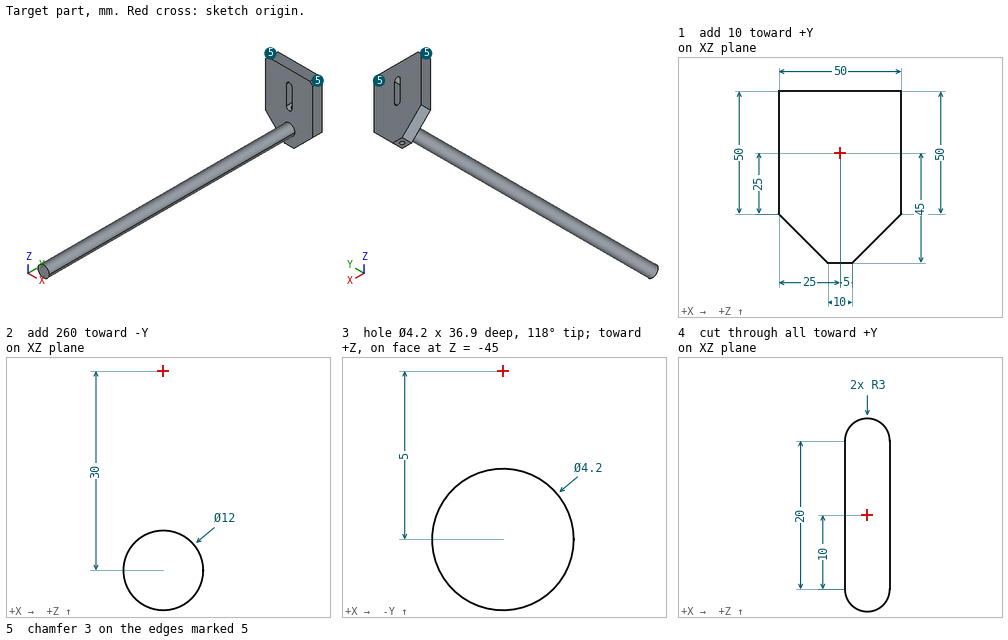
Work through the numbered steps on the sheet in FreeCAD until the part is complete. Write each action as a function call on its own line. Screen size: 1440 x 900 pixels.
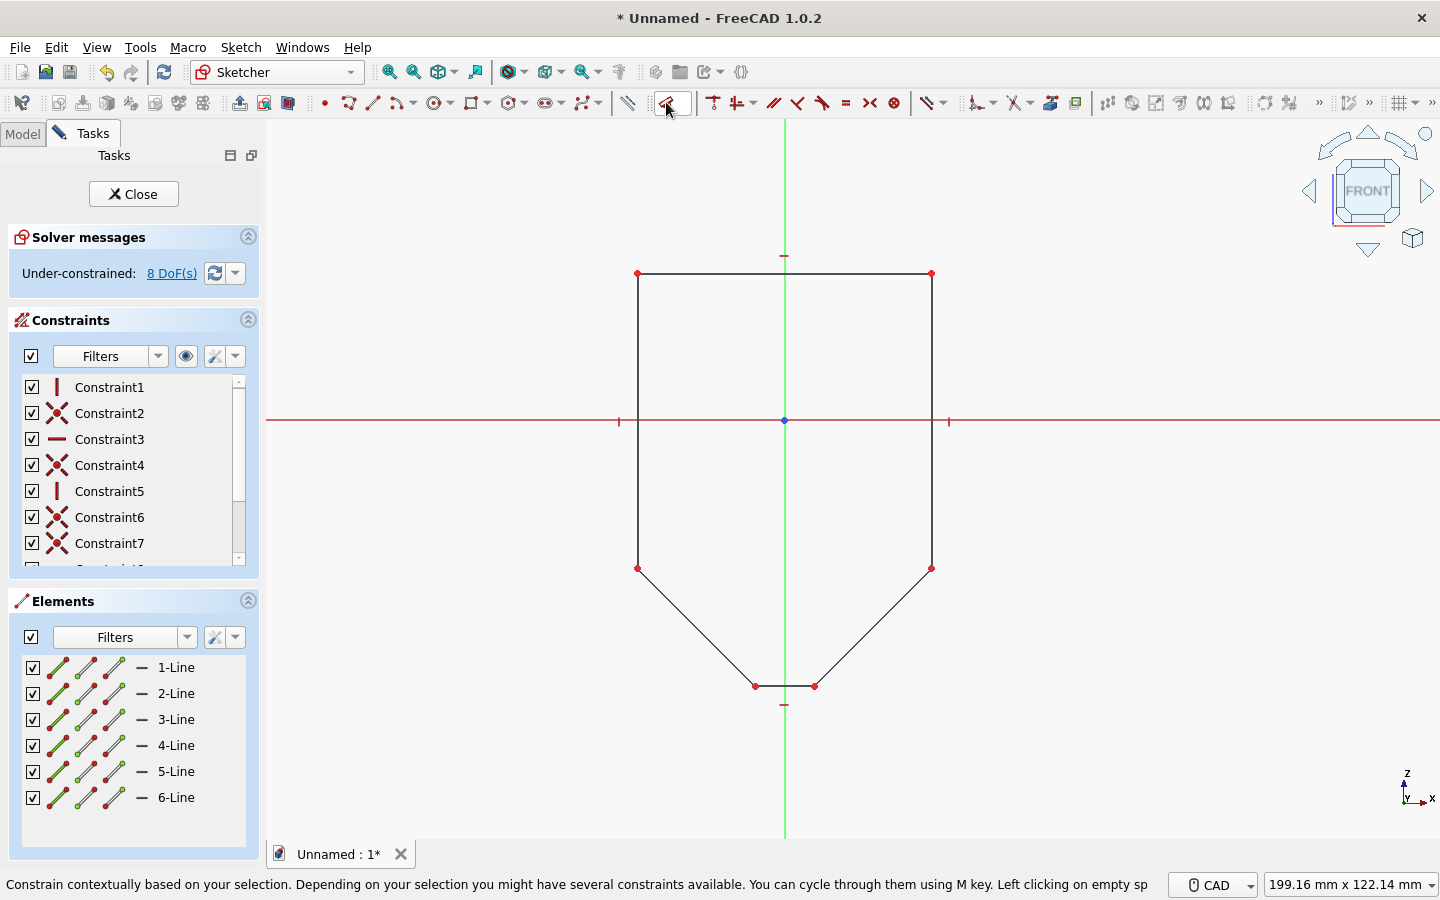
click(638, 480)
click(604, 353)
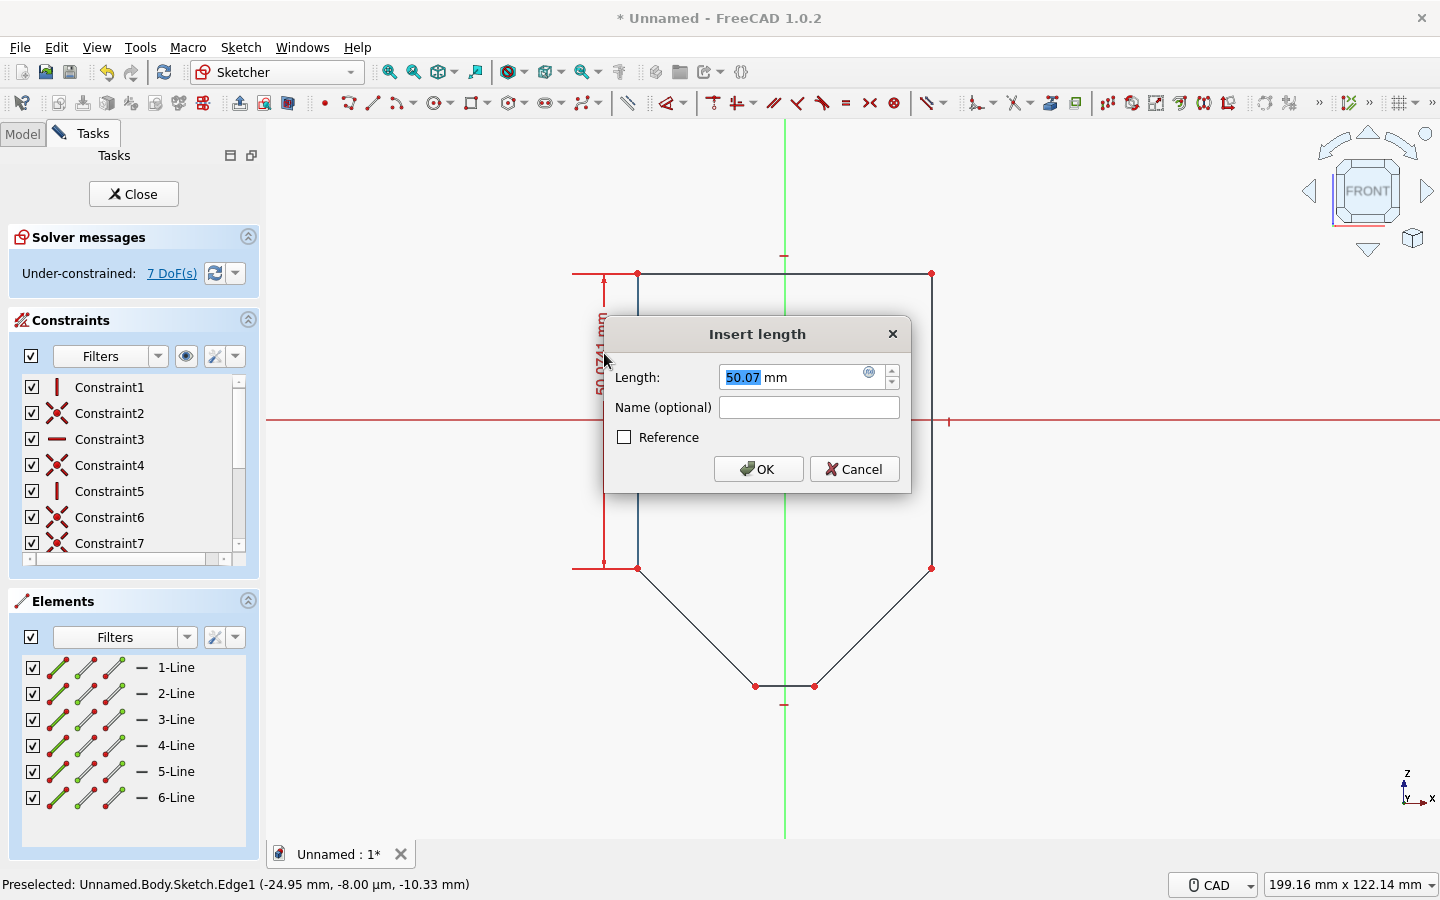
text(50)
key(Return)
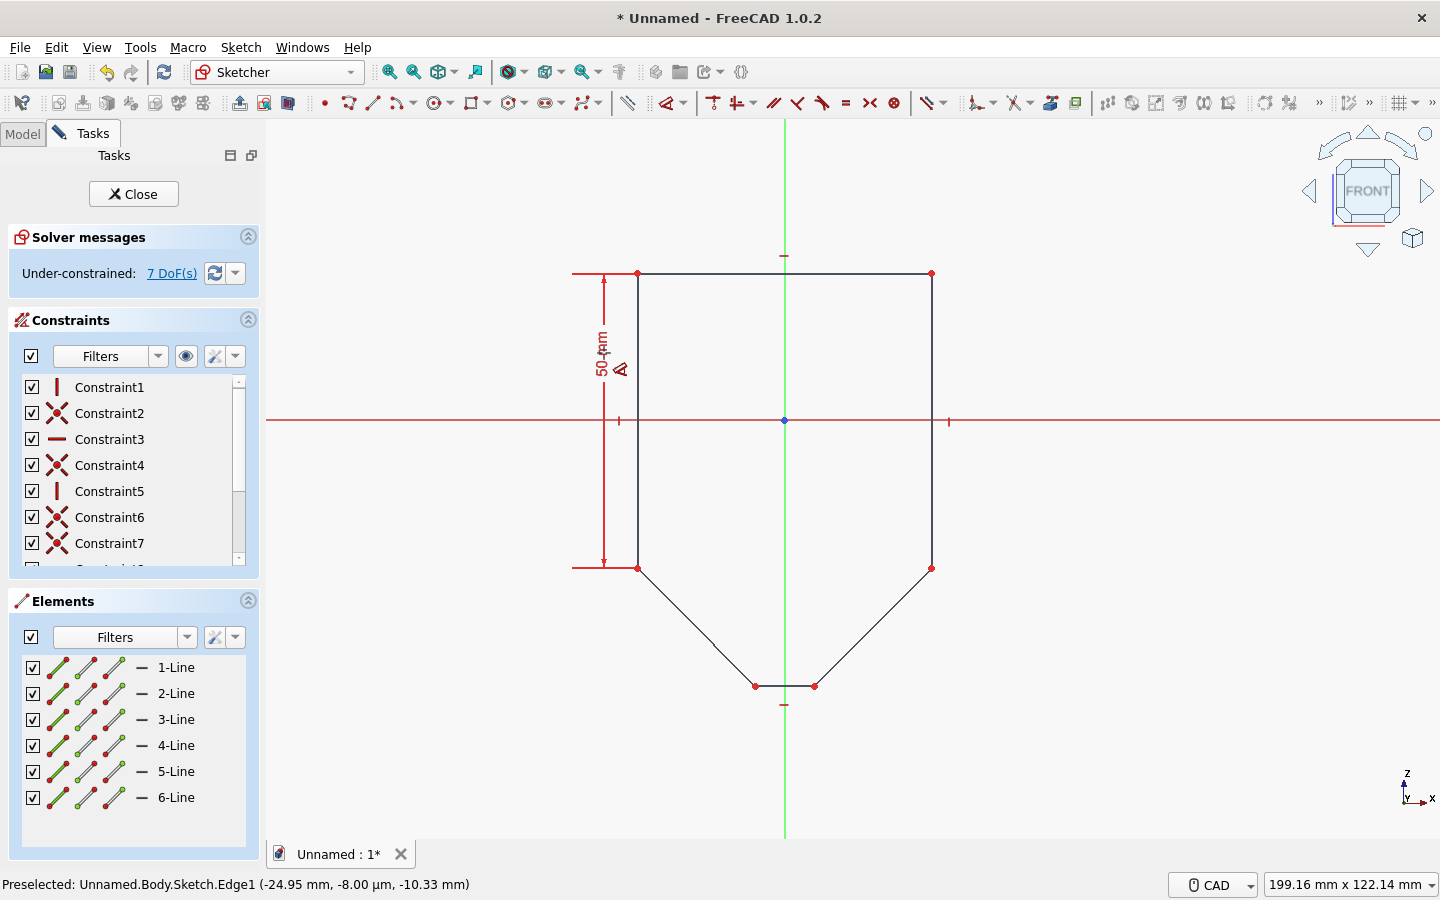
click(726, 274)
click(717, 240)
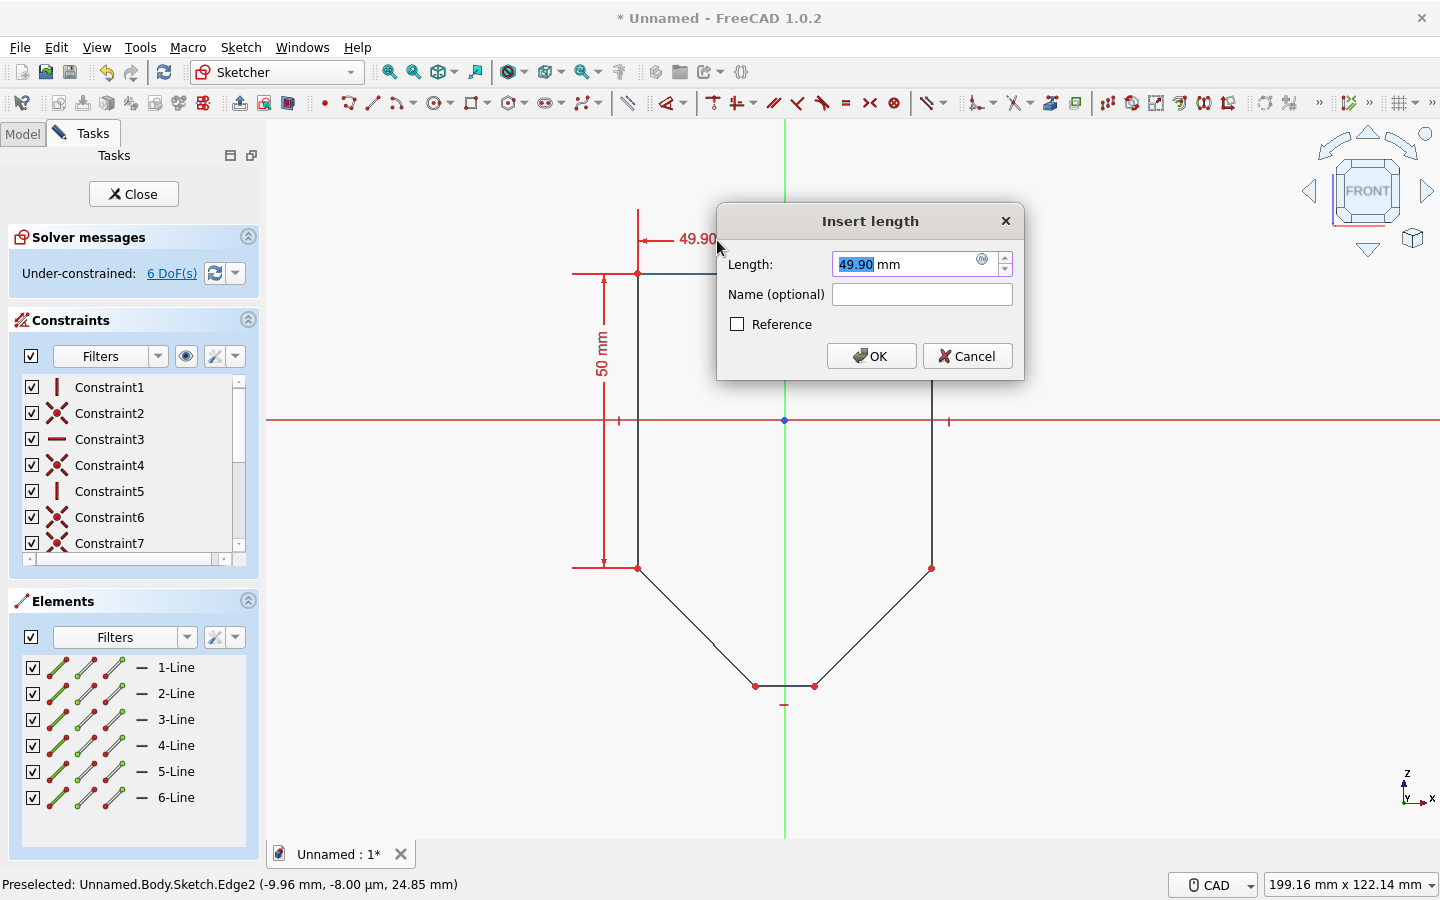
text(50)
key(Return)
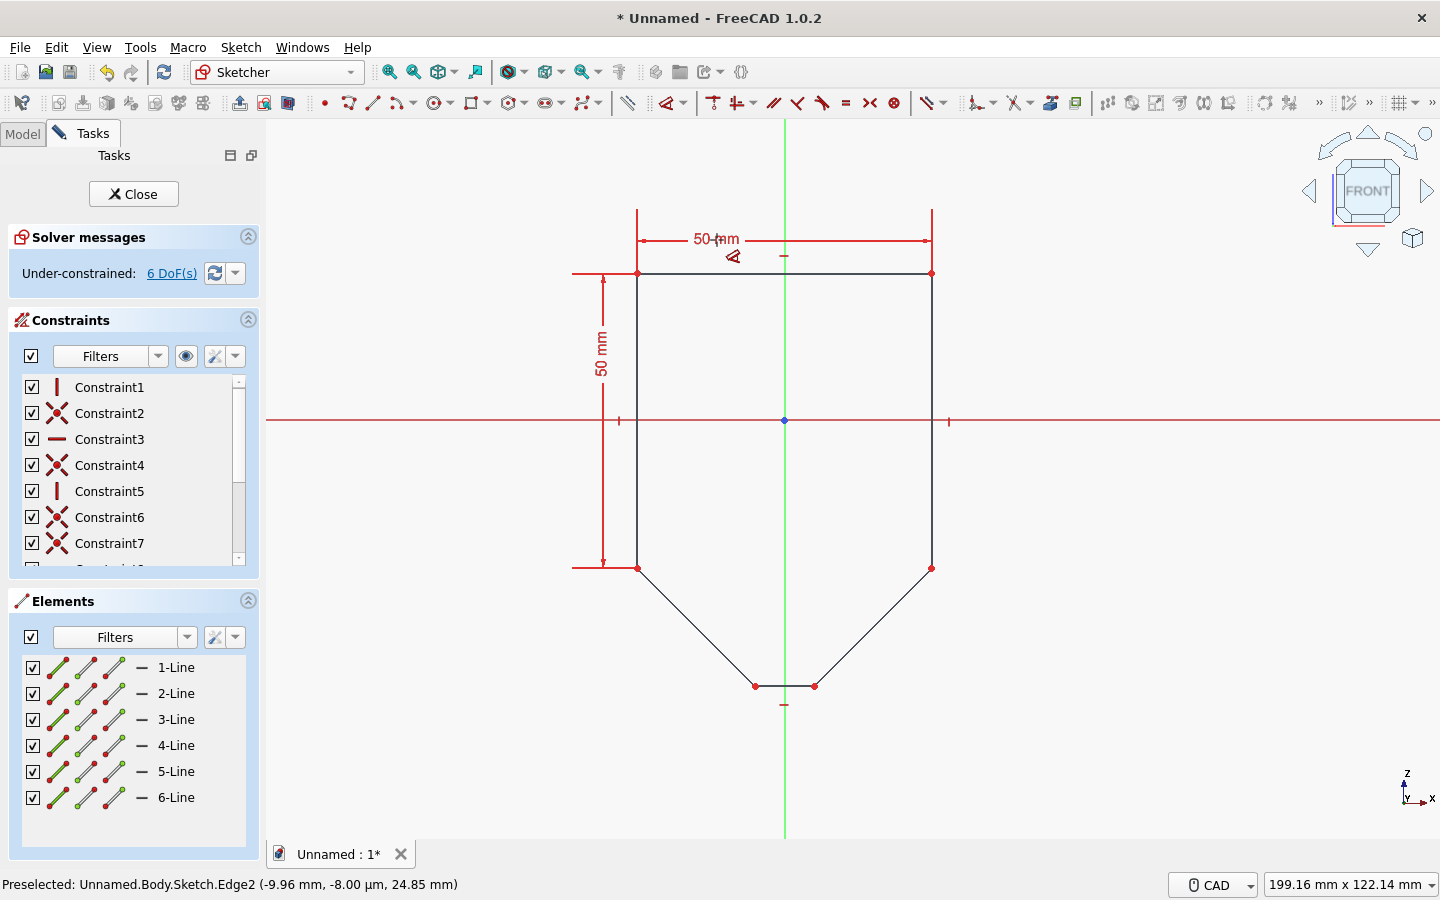
click(932, 362)
click(966, 353)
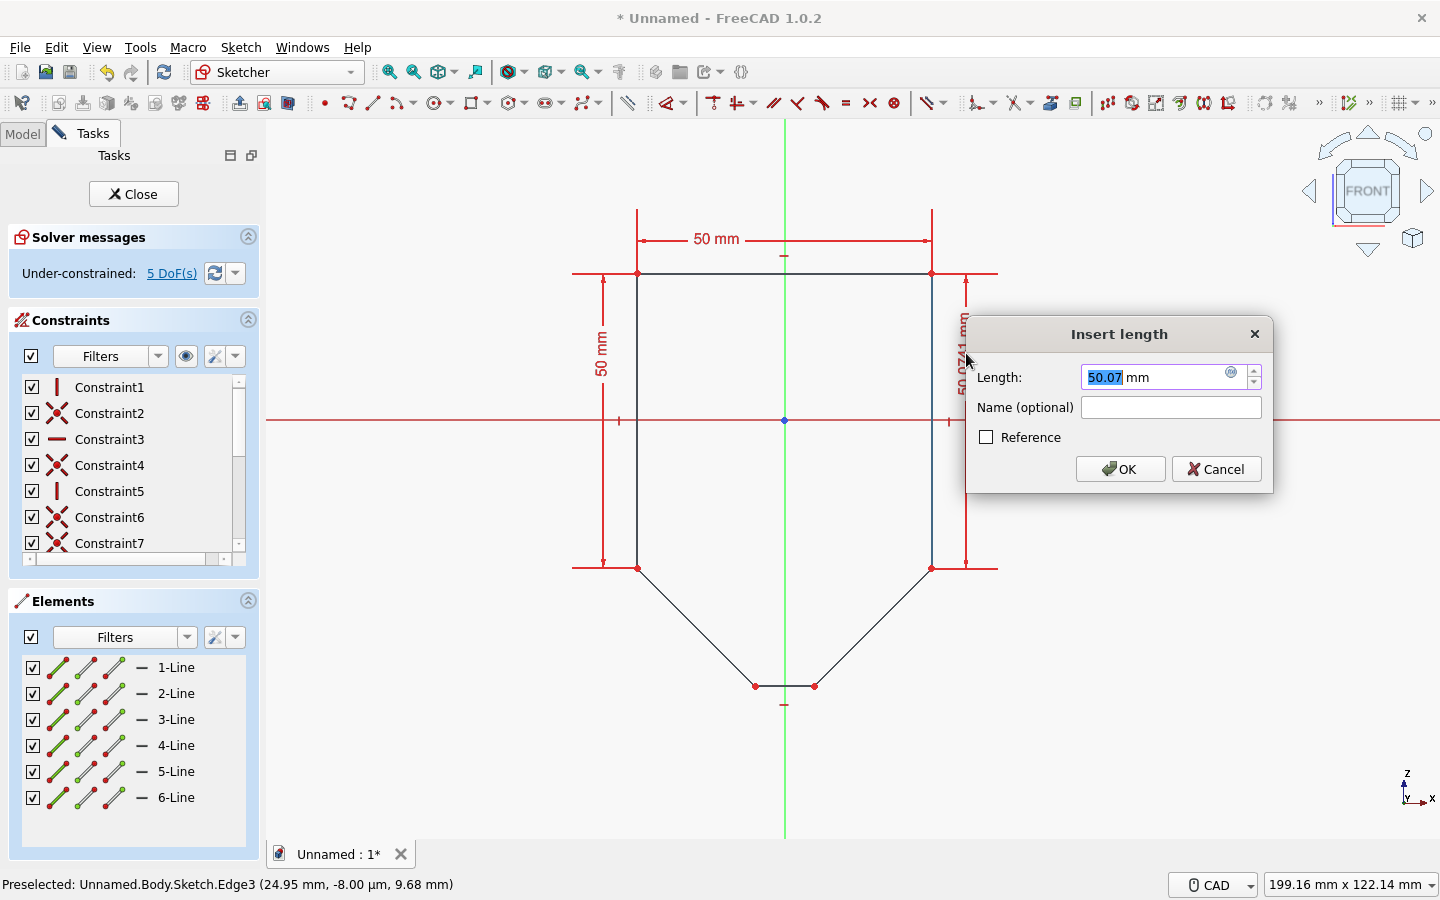
text(50)
key(Return)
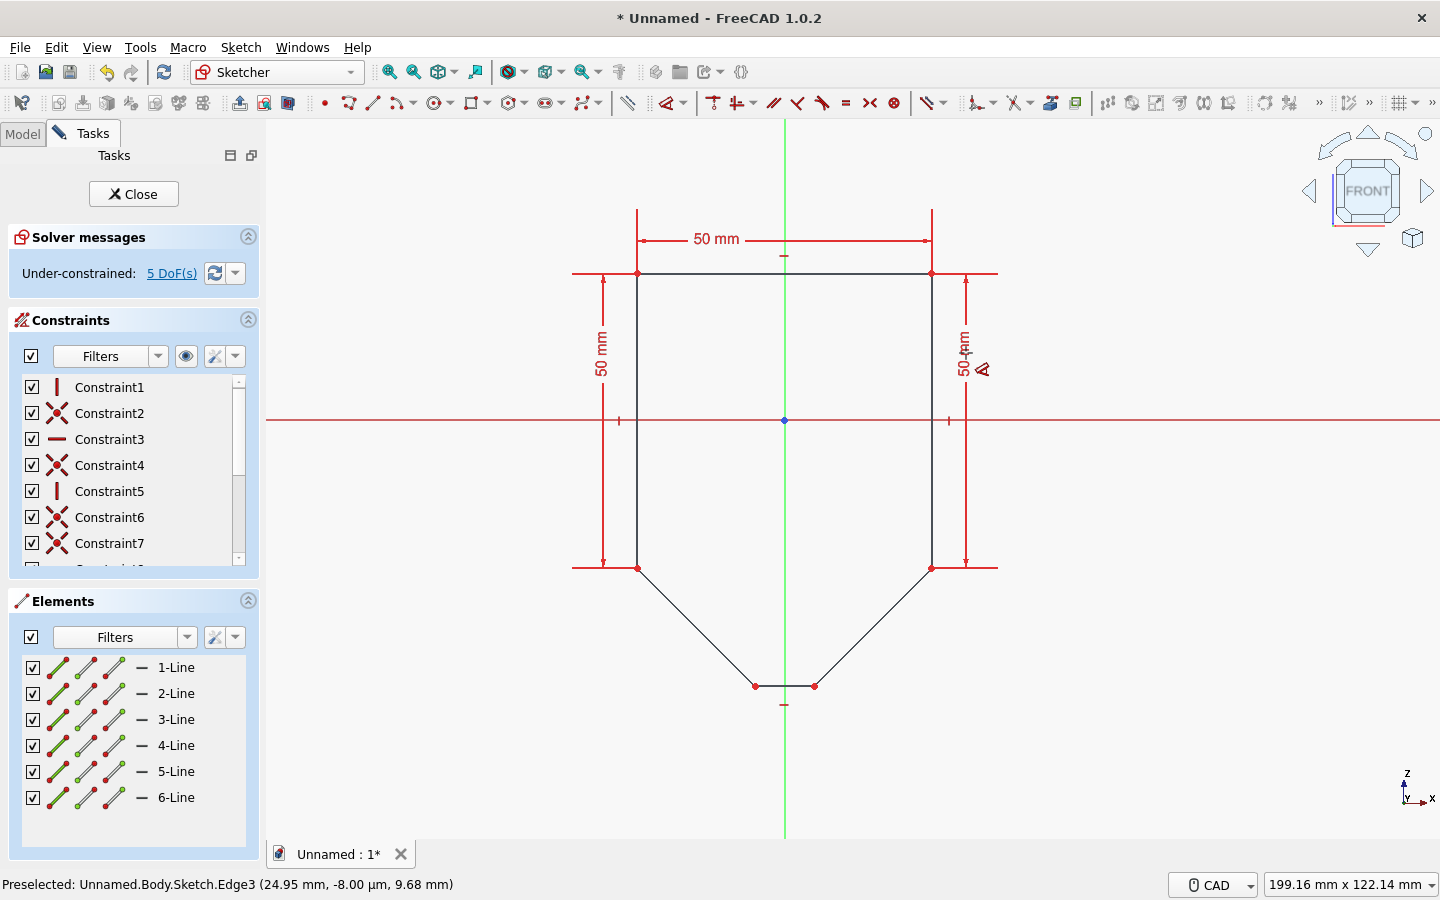
click(796, 686)
click(771, 720)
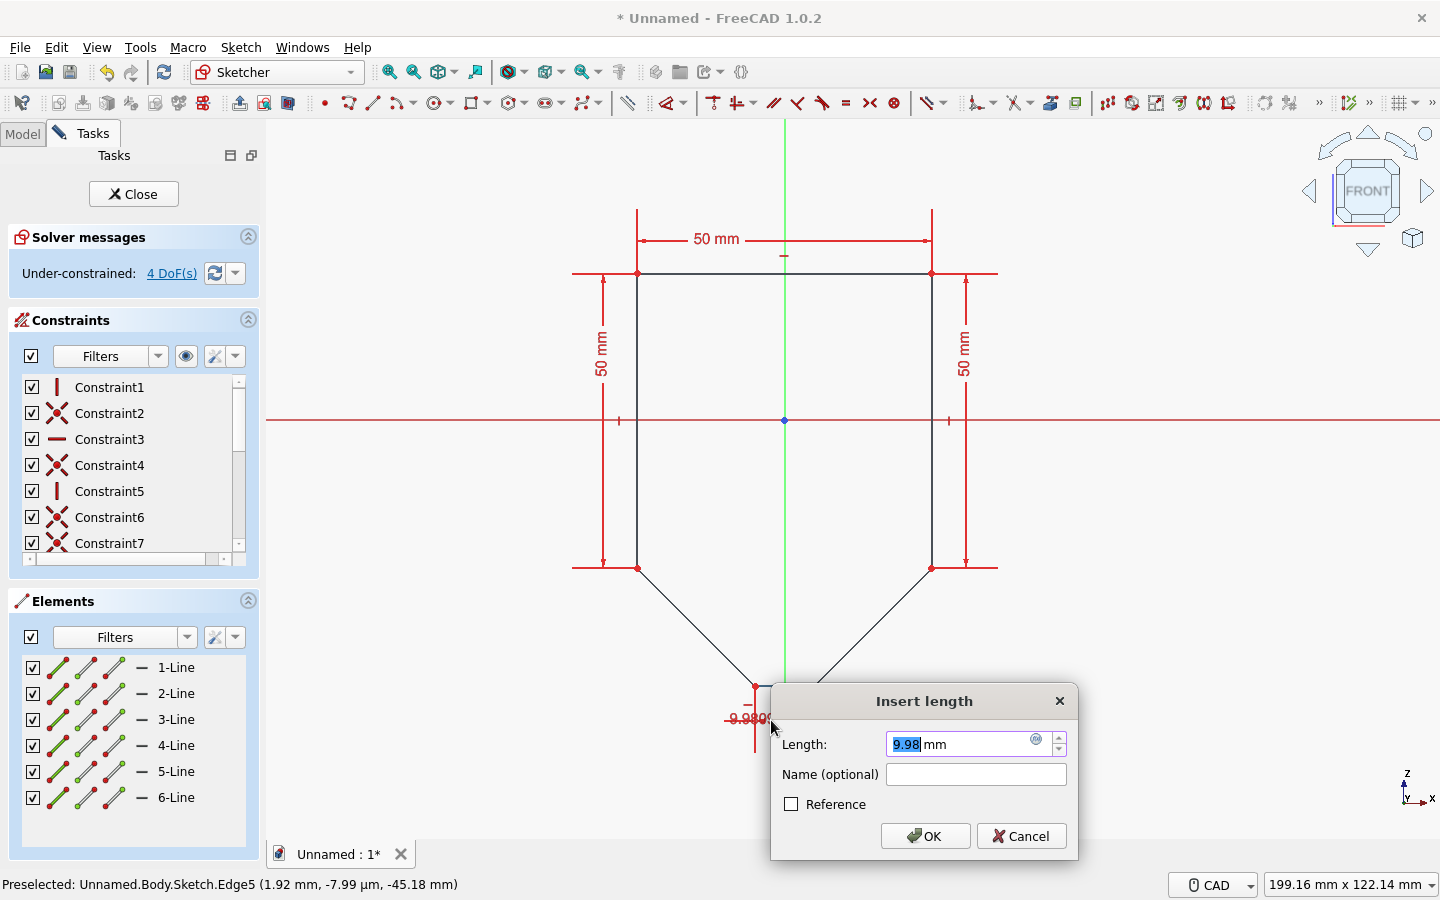
text(10)
key(Return)